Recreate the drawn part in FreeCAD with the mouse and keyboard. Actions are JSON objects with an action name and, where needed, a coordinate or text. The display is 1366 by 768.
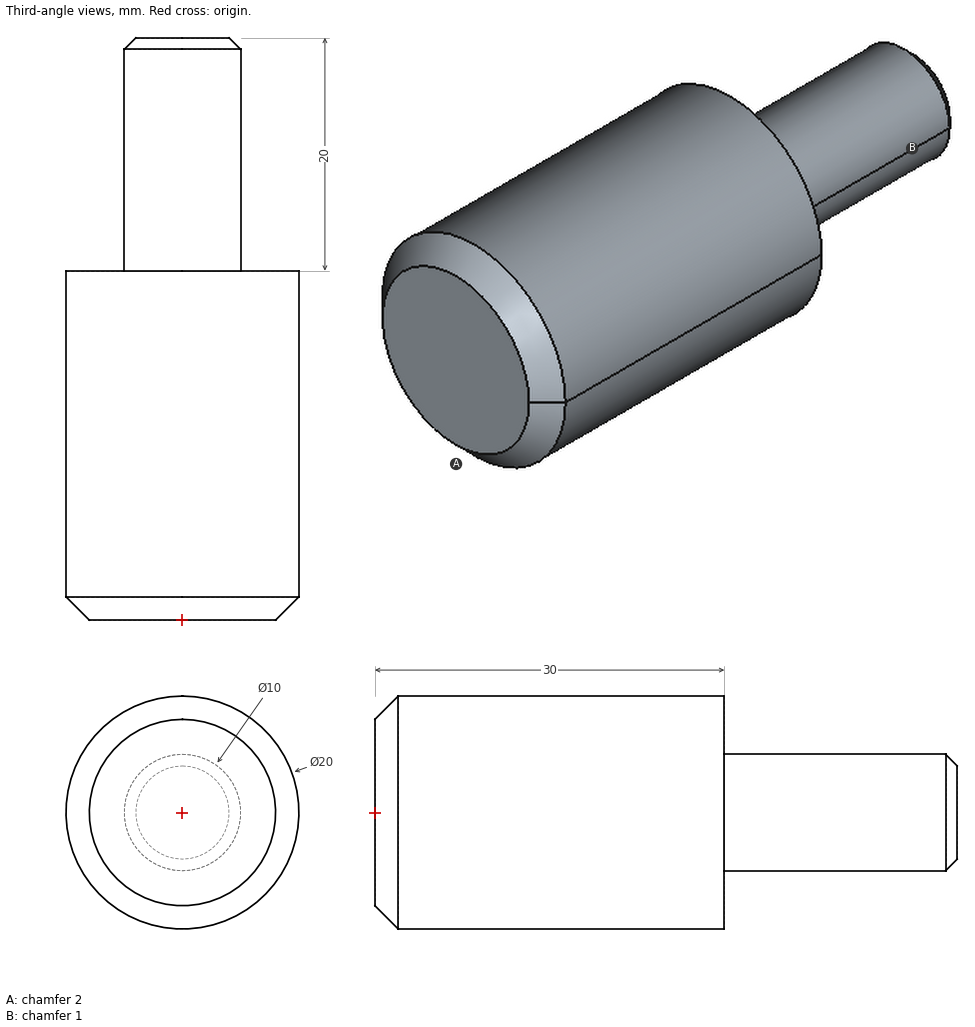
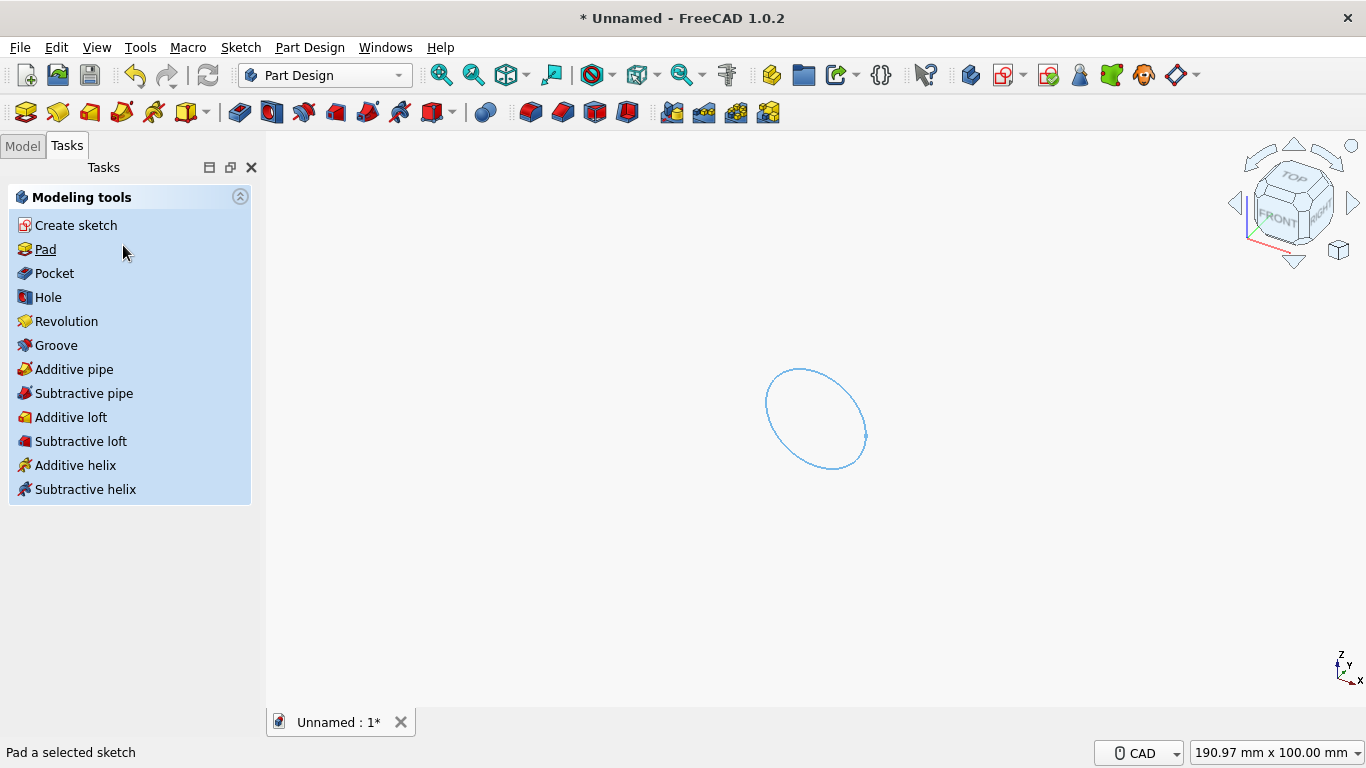
{"action": "left_click", "coordinate": [26, 112]}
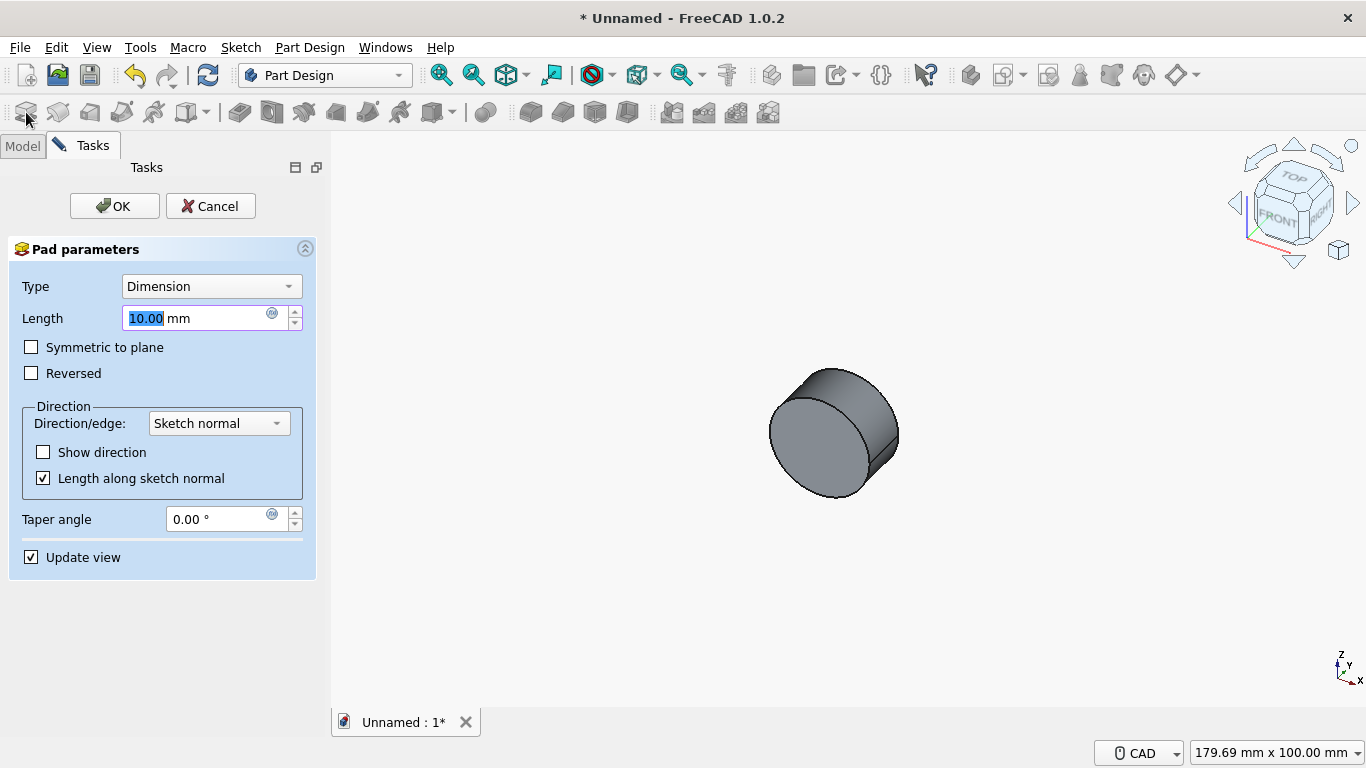
{"action": "type", "text": "30"}
{"action": "key", "text": "Tab"}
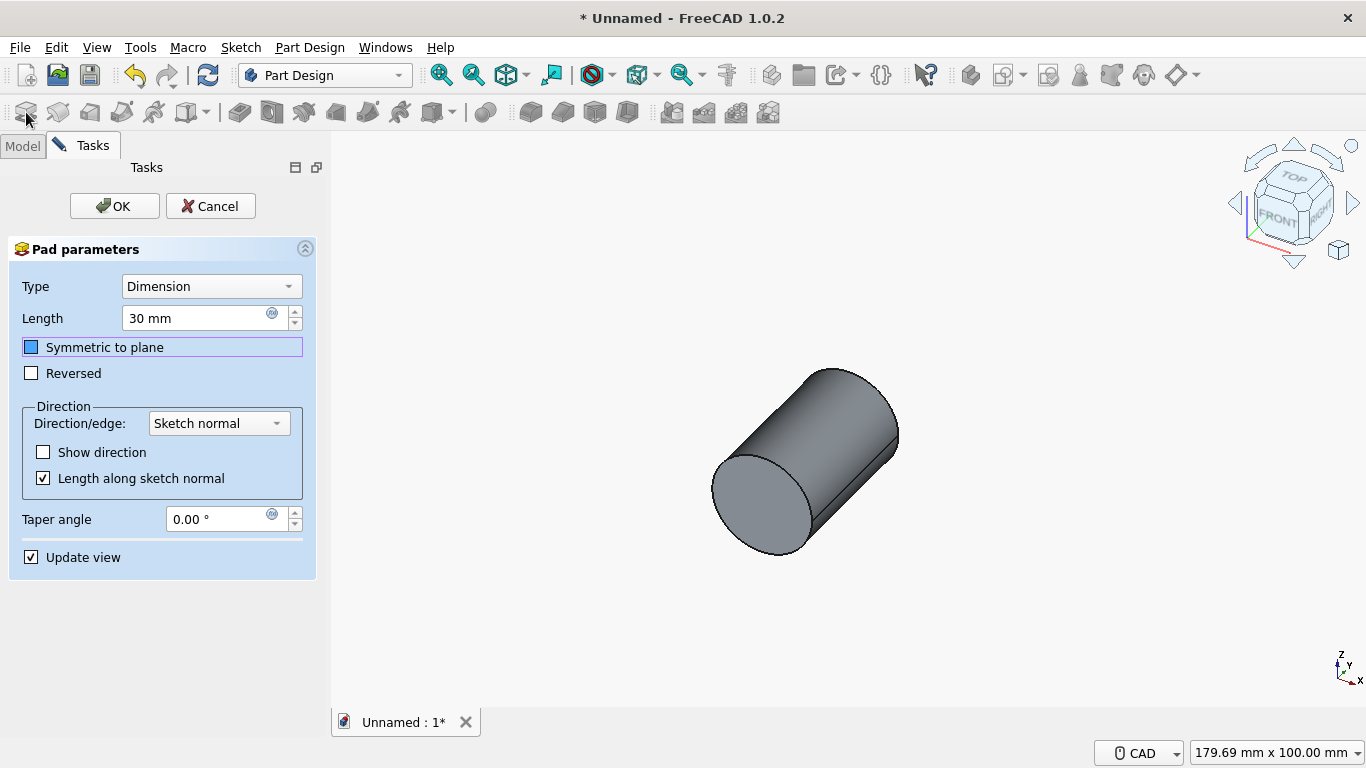
{"action": "left_click", "coordinate": [30, 373]}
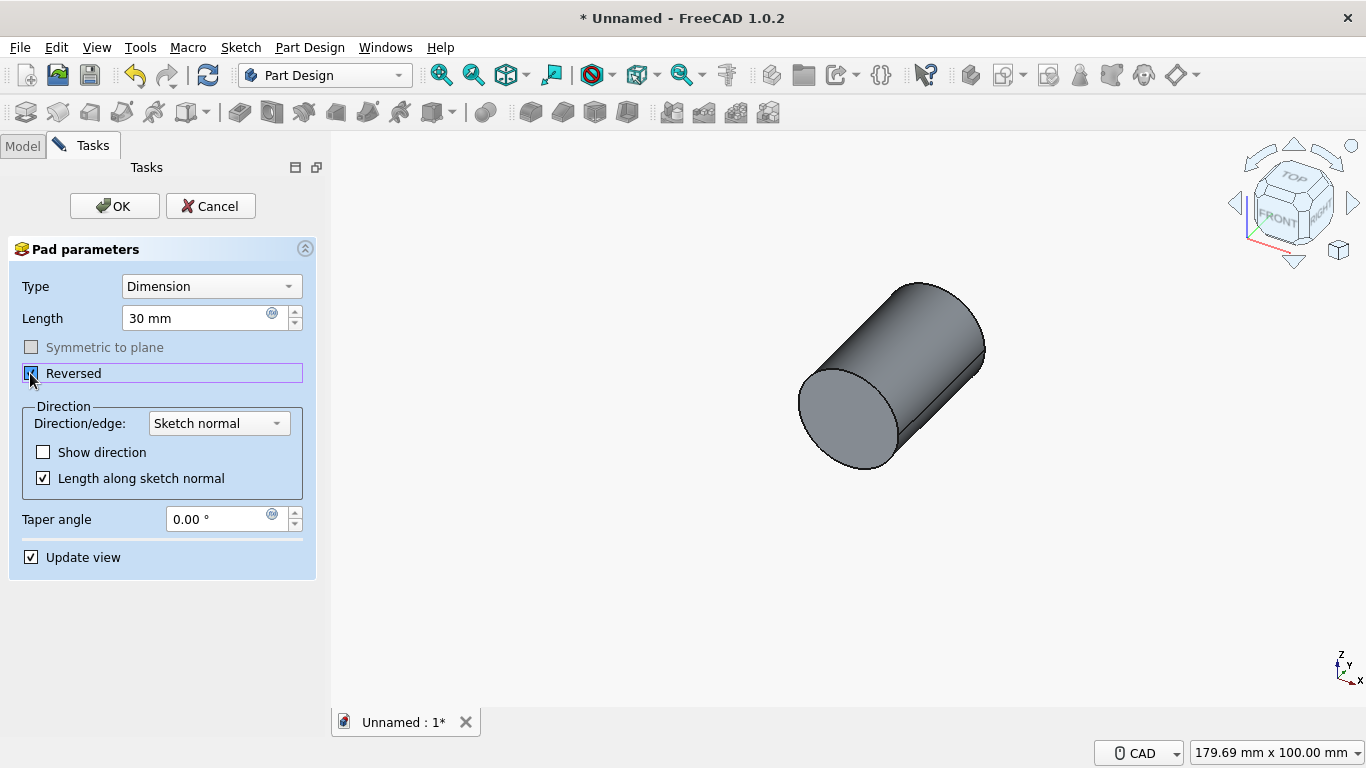
{"action": "left_click", "coordinate": [115, 206]}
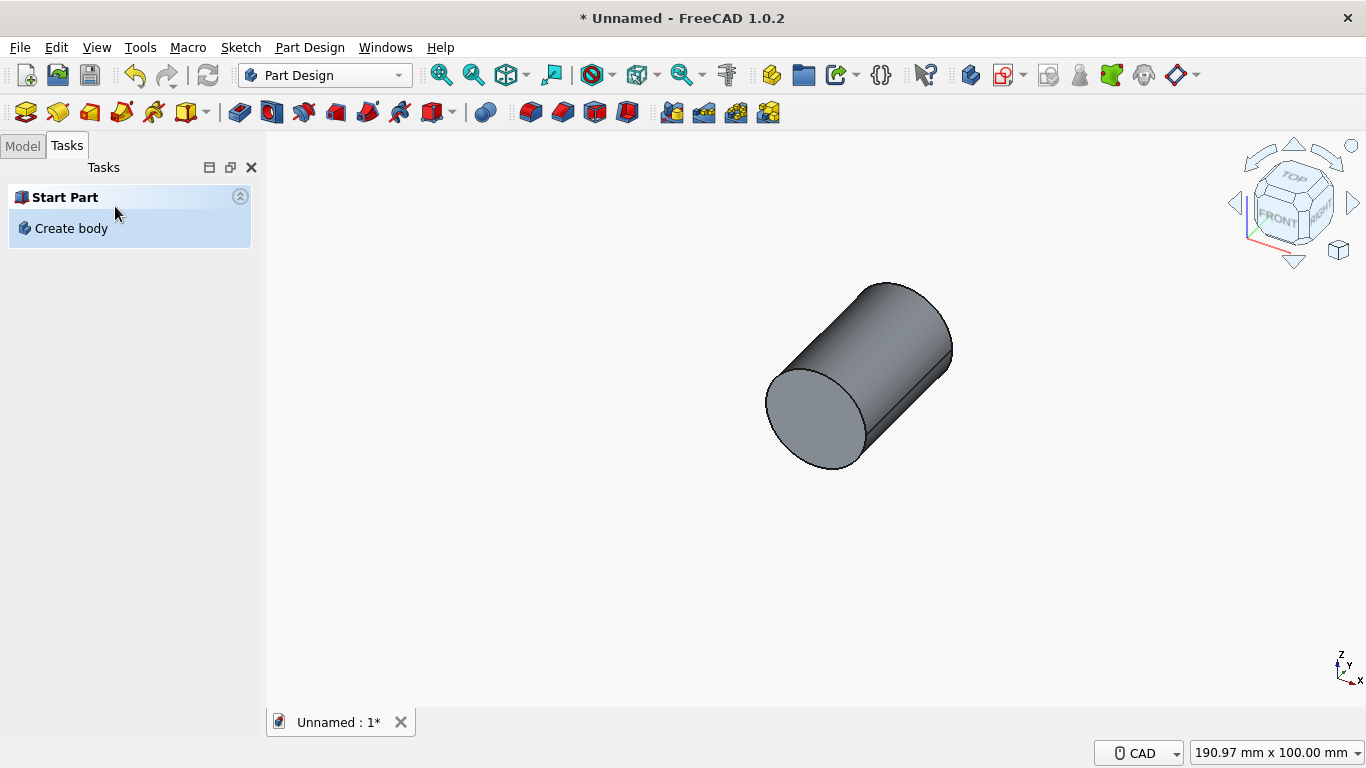
{"action": "left_click", "coordinate": [442, 76]}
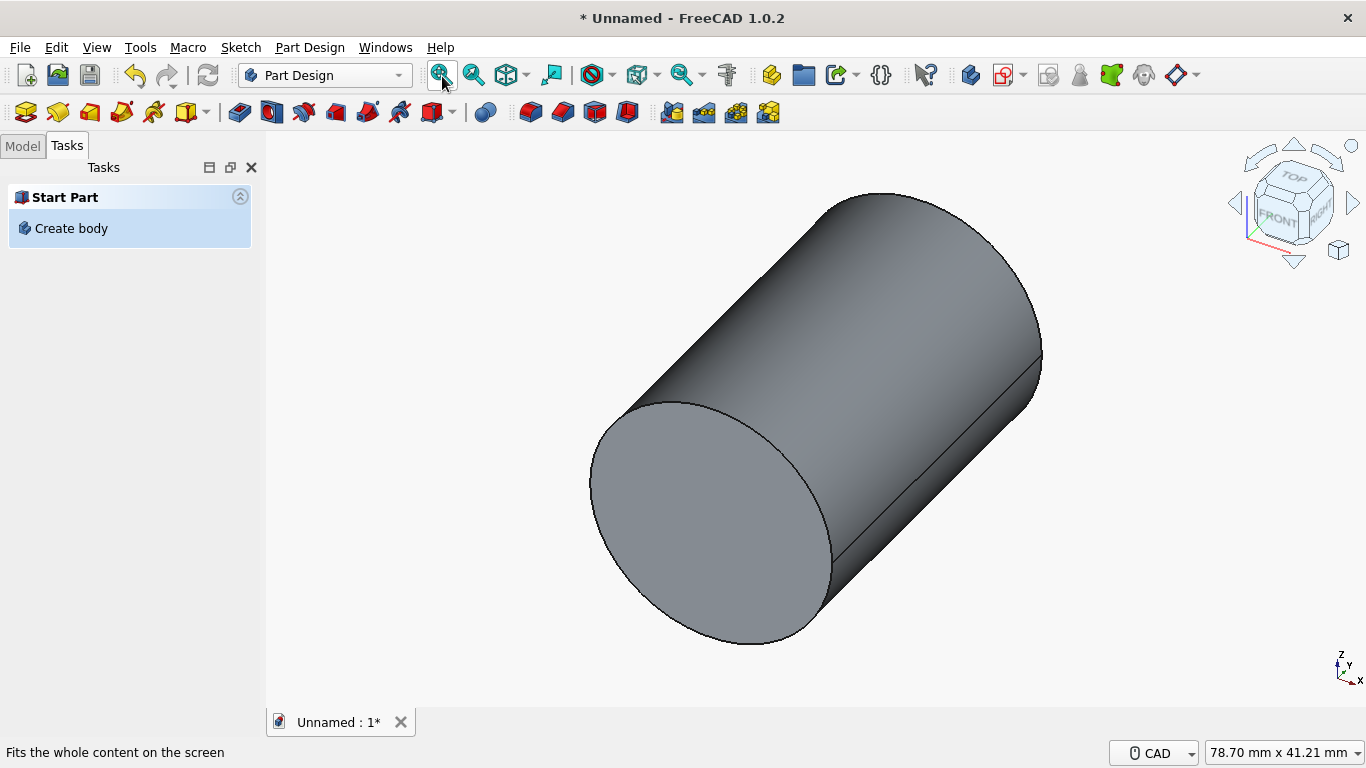
{"action": "key", "text": "4"}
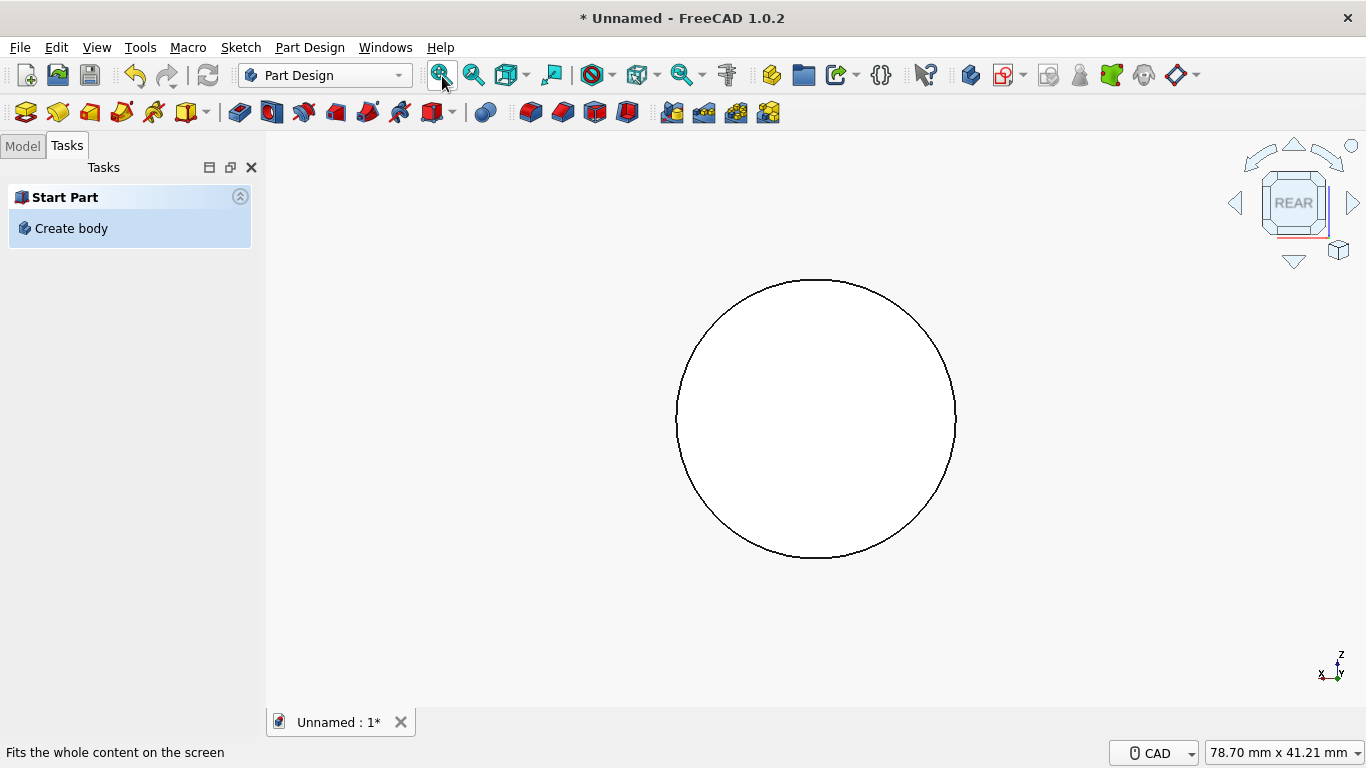
{"action": "left_click", "coordinate": [816, 418]}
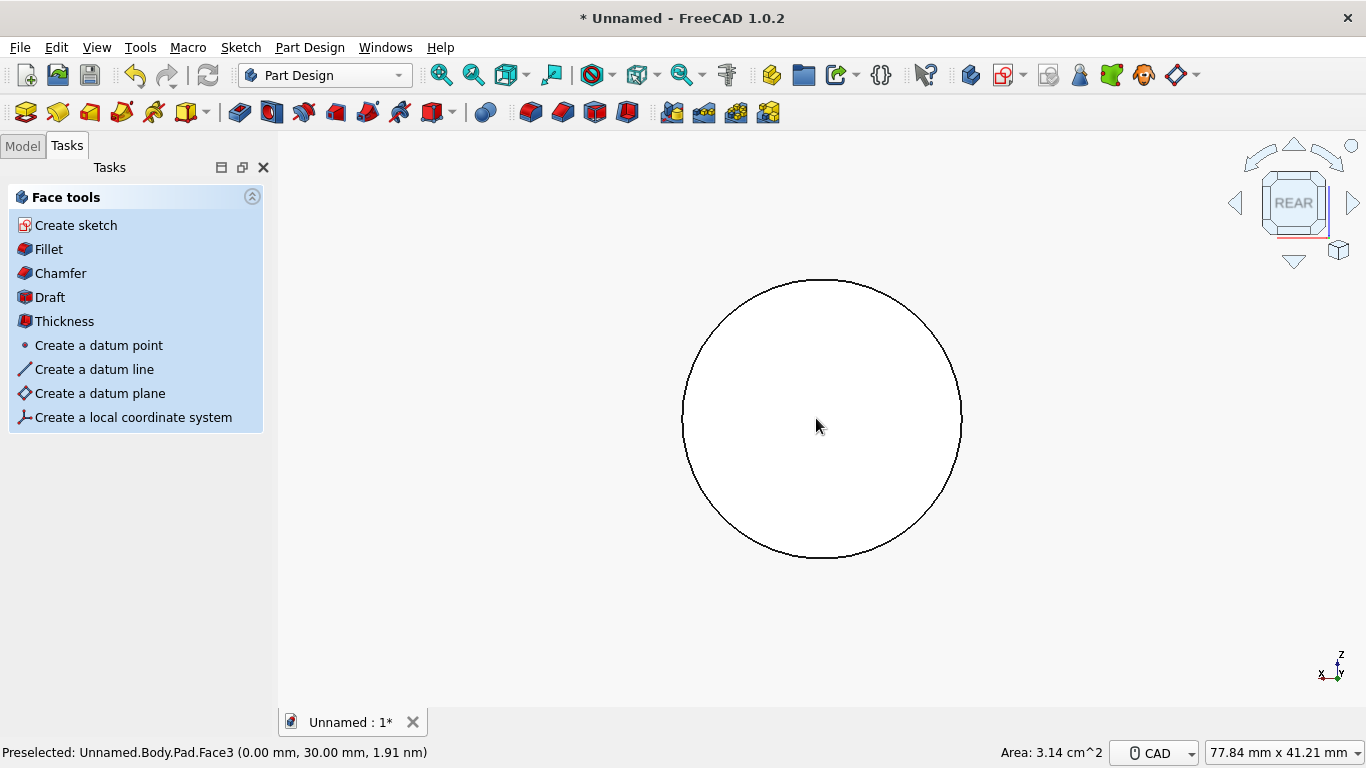
{"action": "left_click", "coordinate": [1004, 76]}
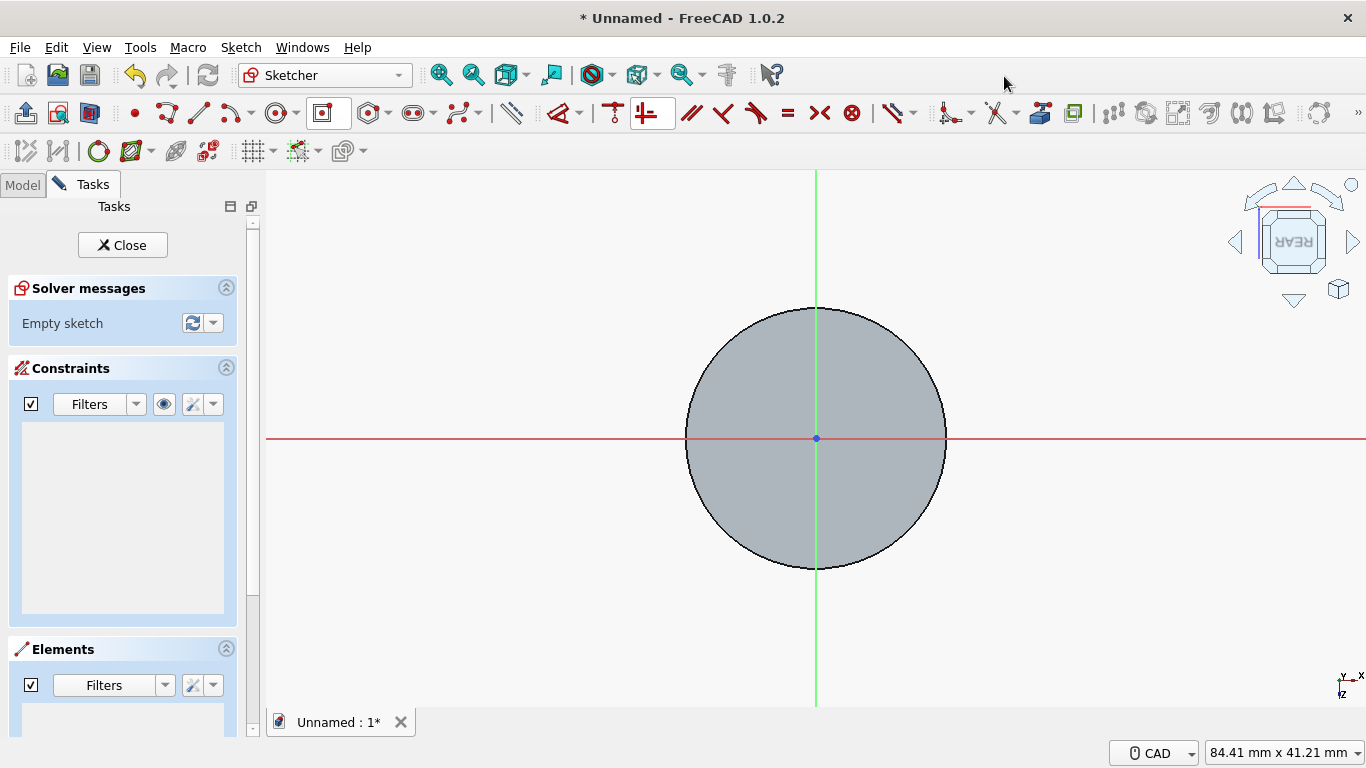
{"action": "scroll", "coordinate": [856, 438], "scroll_direction": "up", "scroll_amount": 5}